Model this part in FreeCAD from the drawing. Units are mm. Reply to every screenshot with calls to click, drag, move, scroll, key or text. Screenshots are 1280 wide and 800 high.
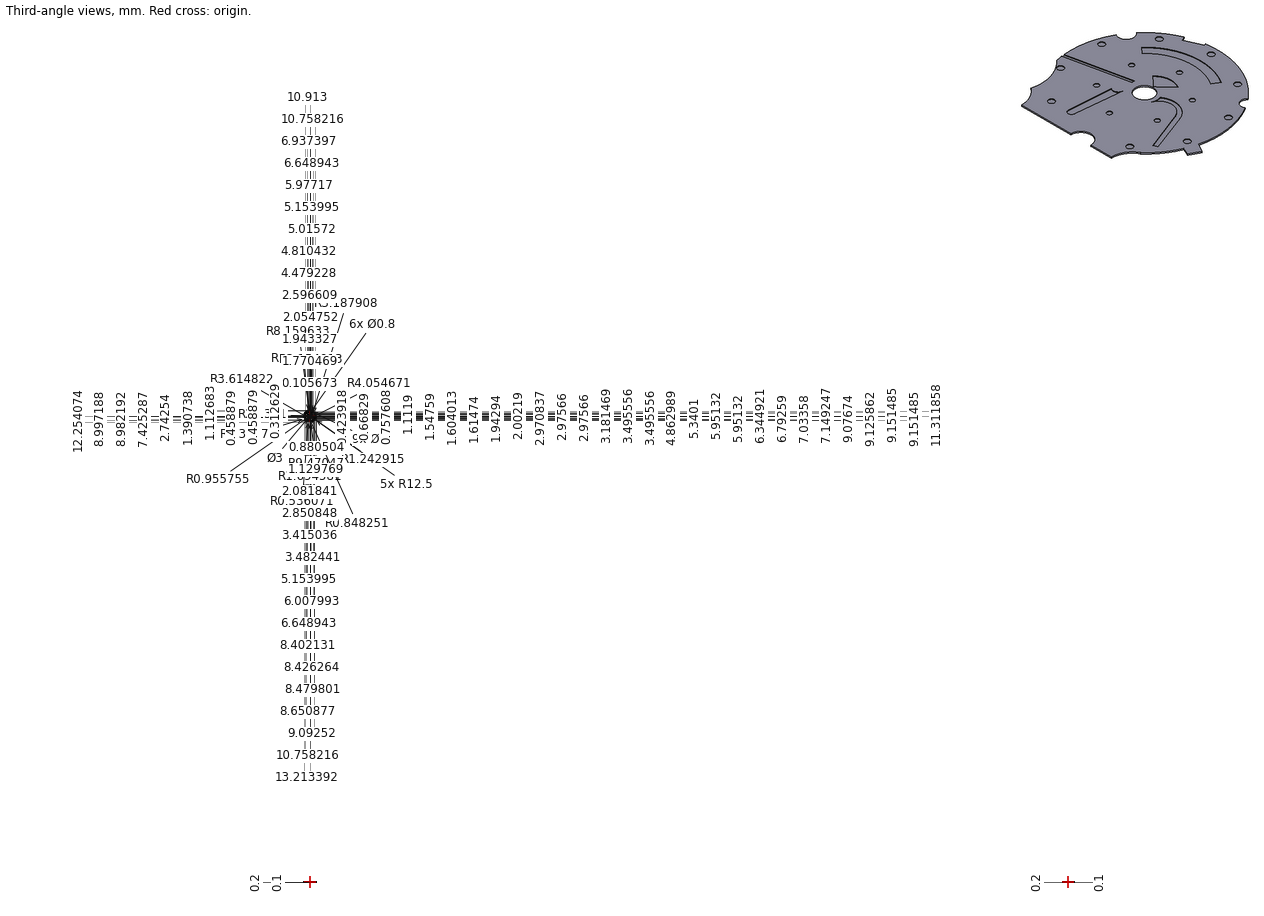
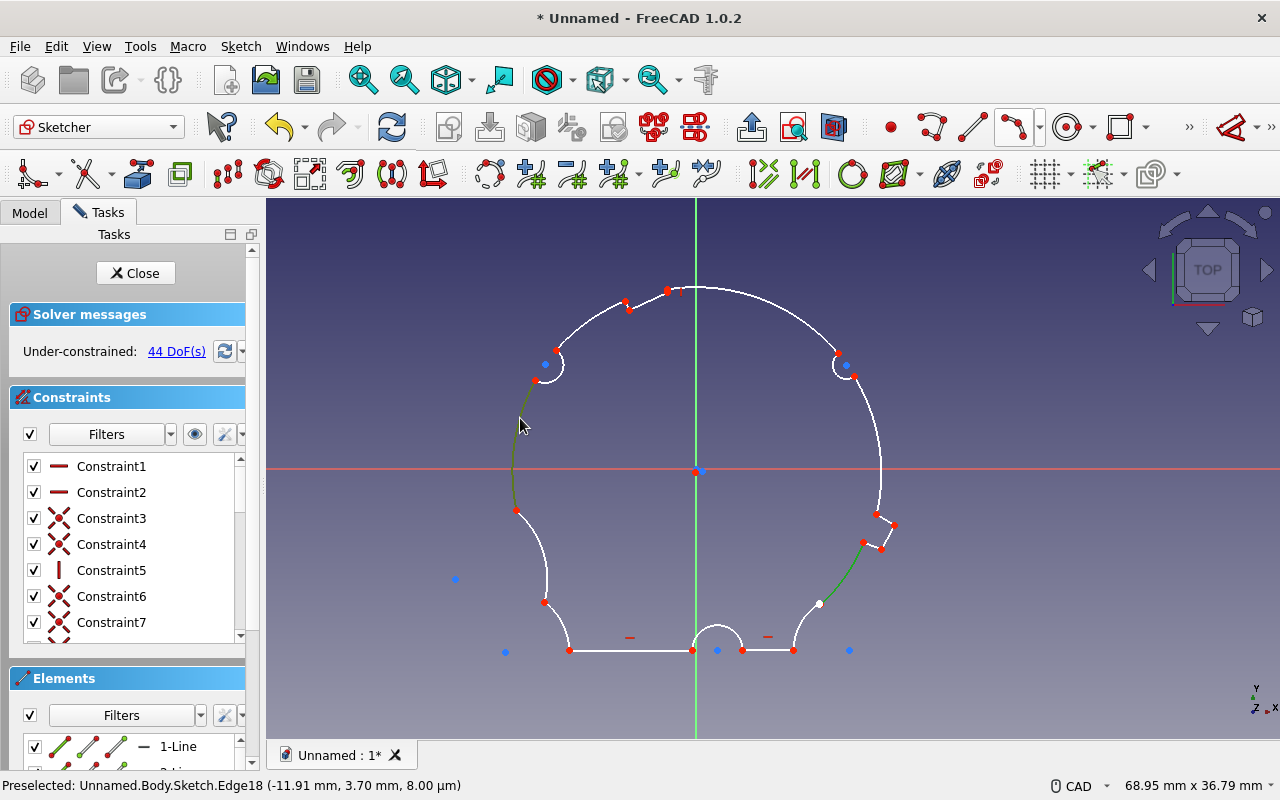
key(c)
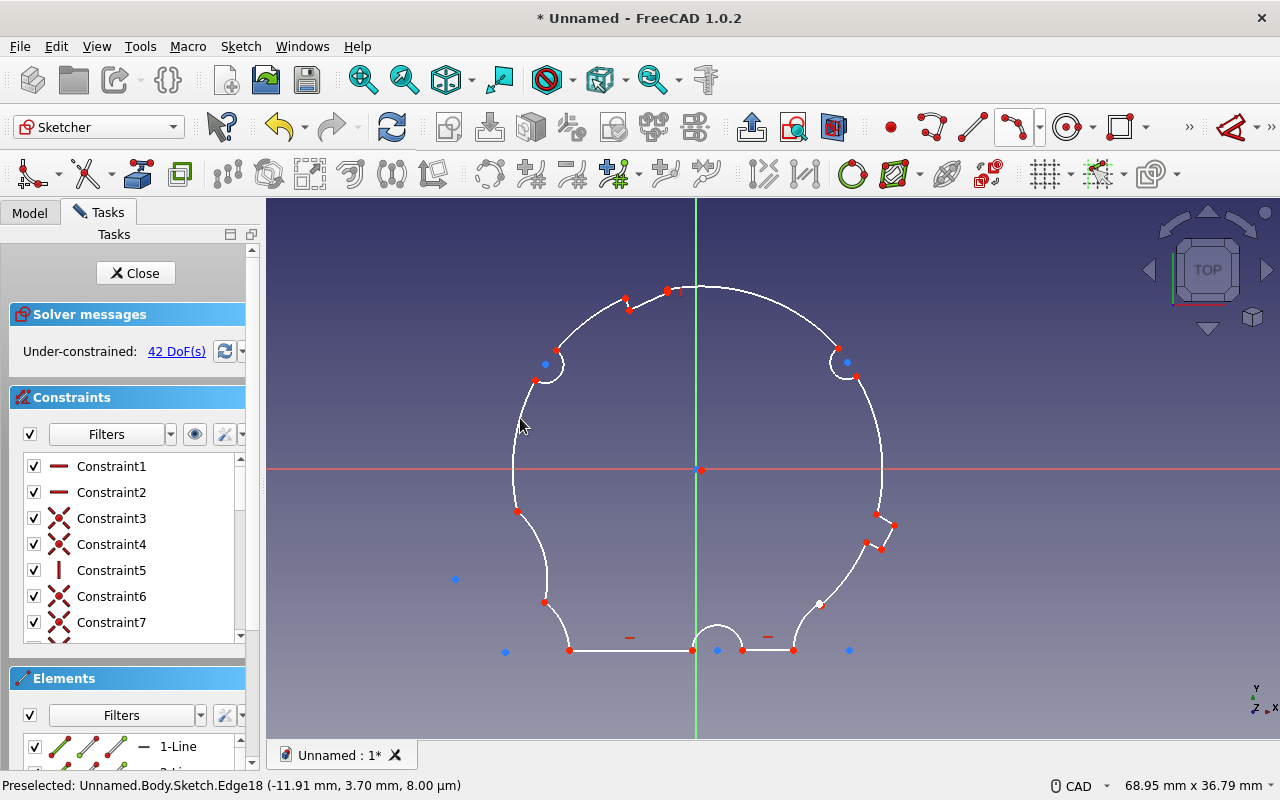
scroll(699, 470, up, 5)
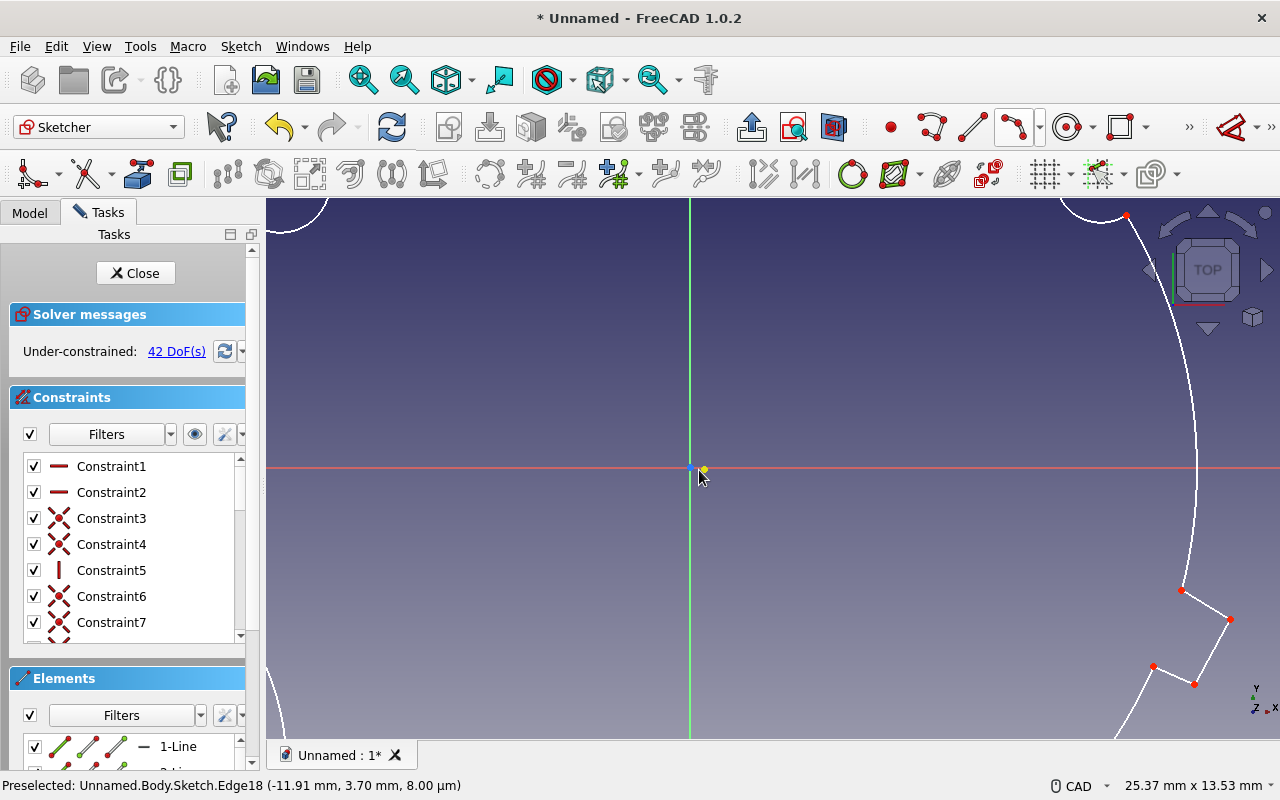
drag(680, 458, 715, 479)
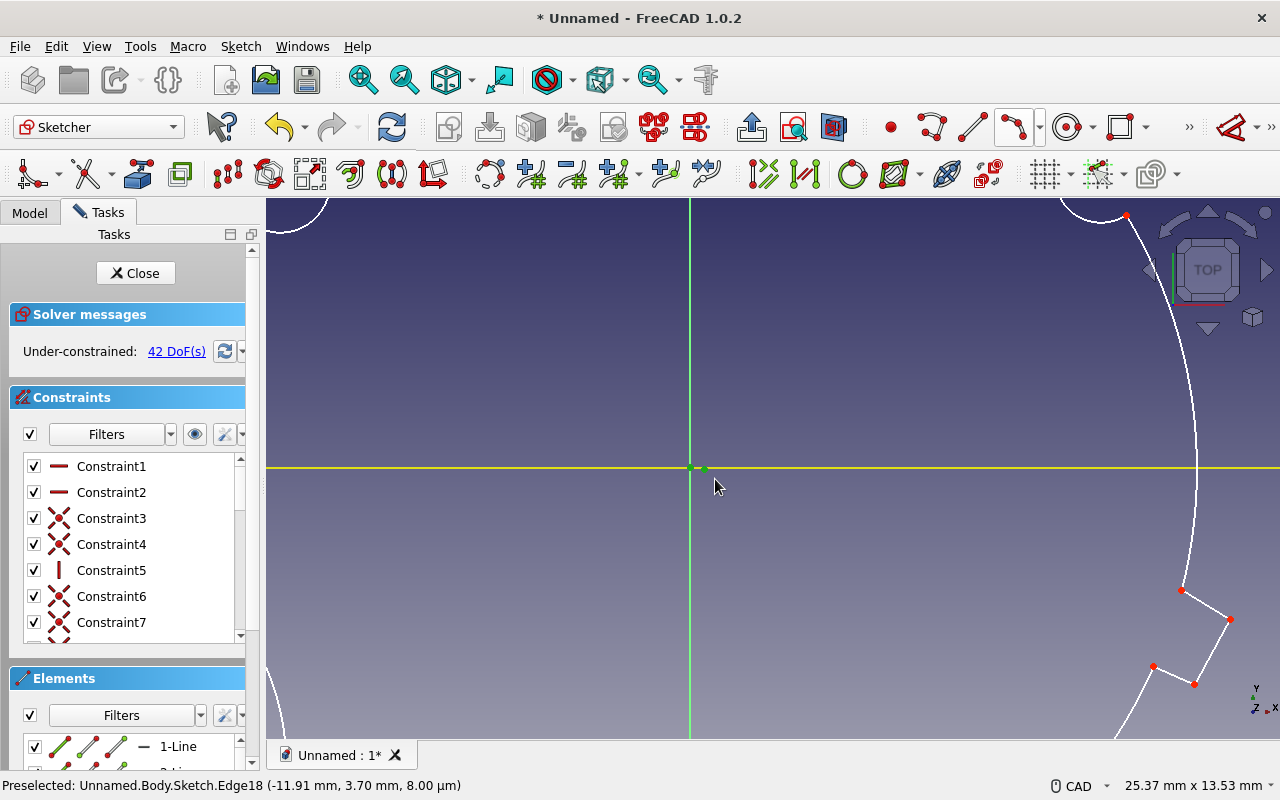
key(c)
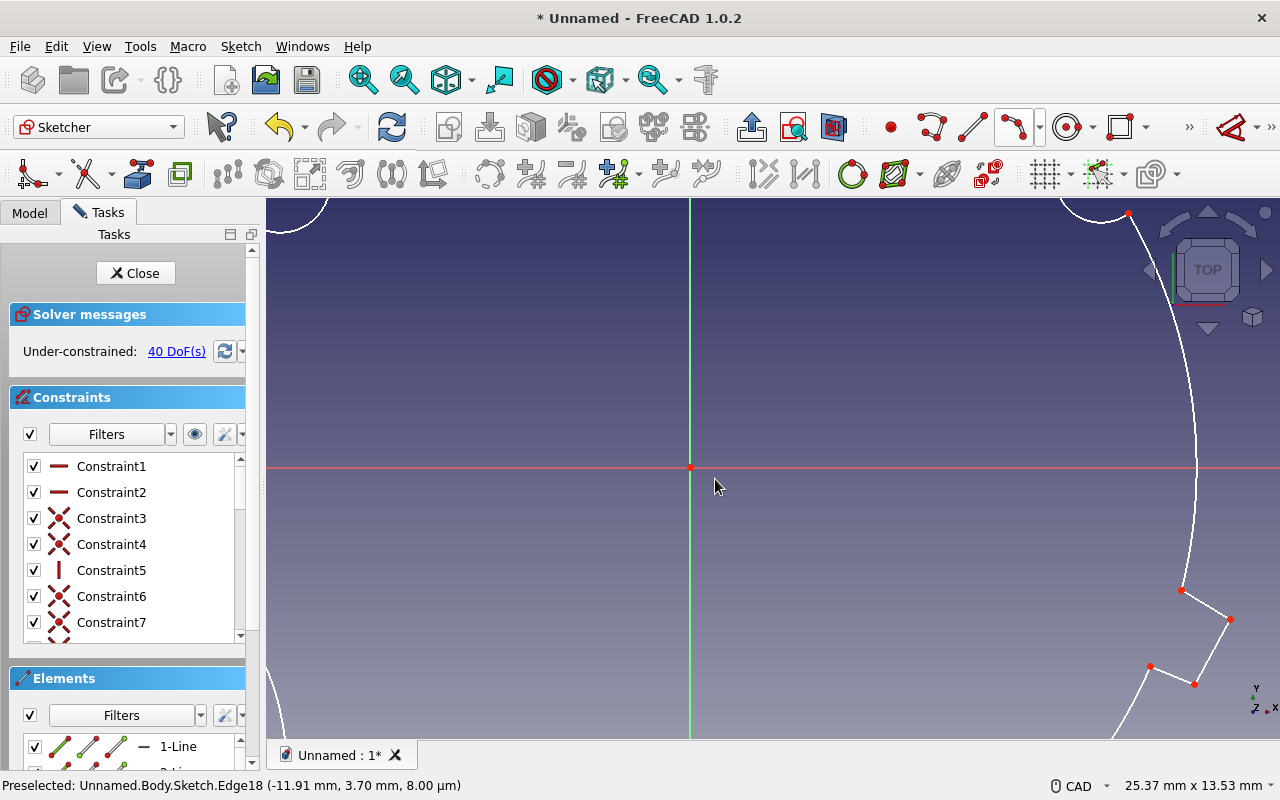
scroll(699, 470, down, 5)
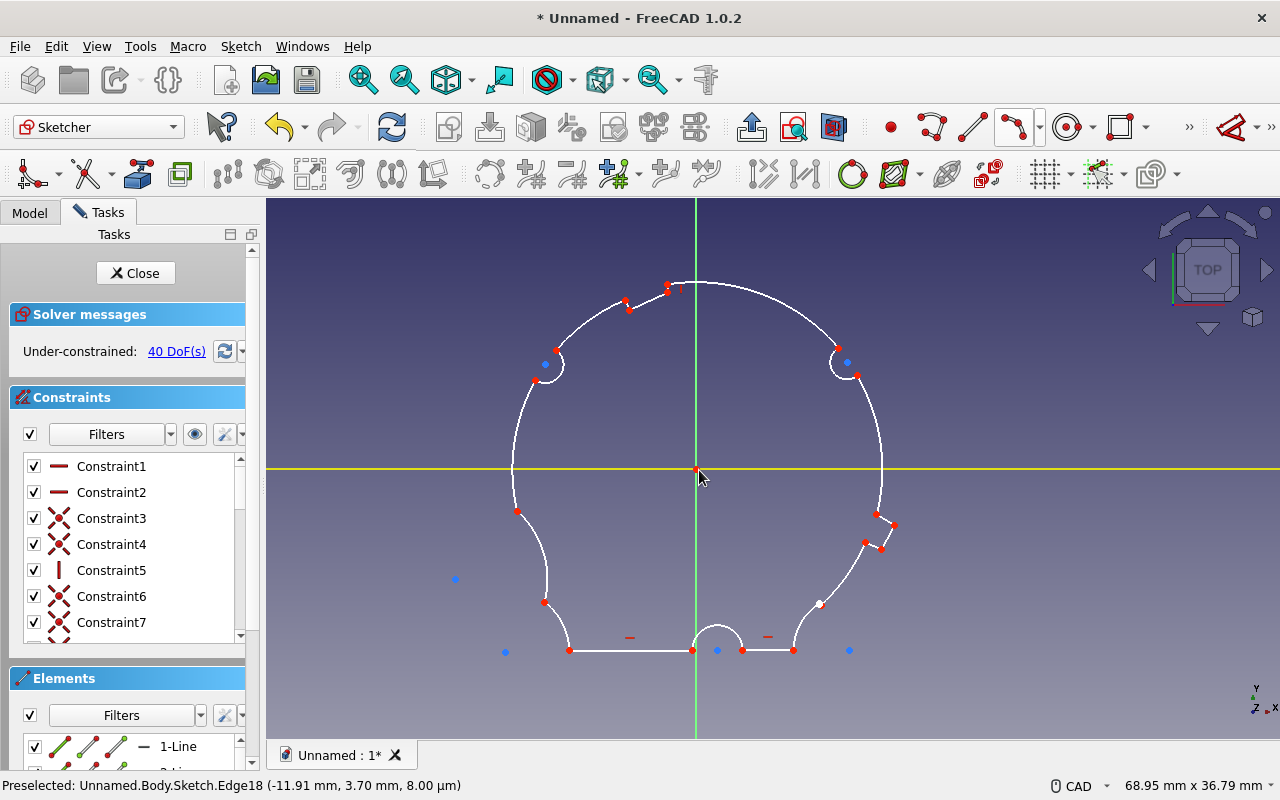
click(837, 588)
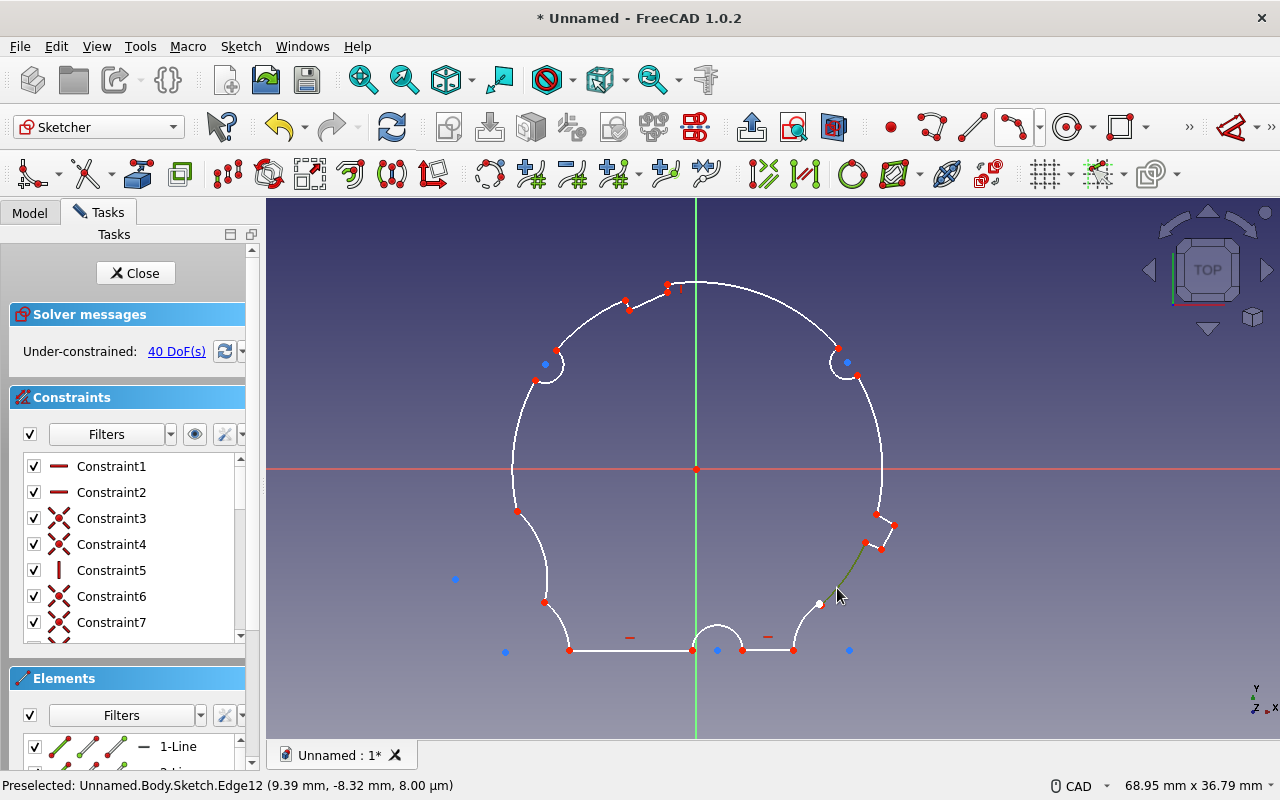
click(882, 472)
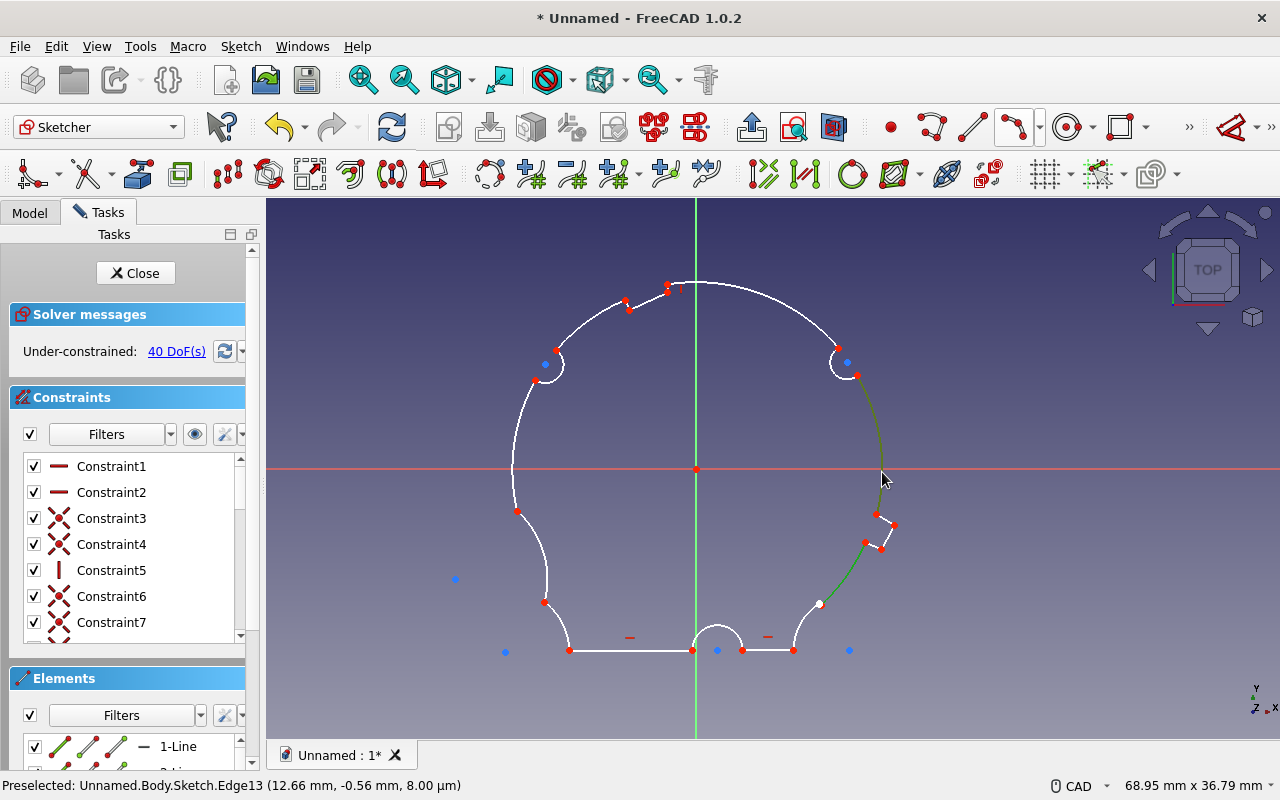
click(795, 311)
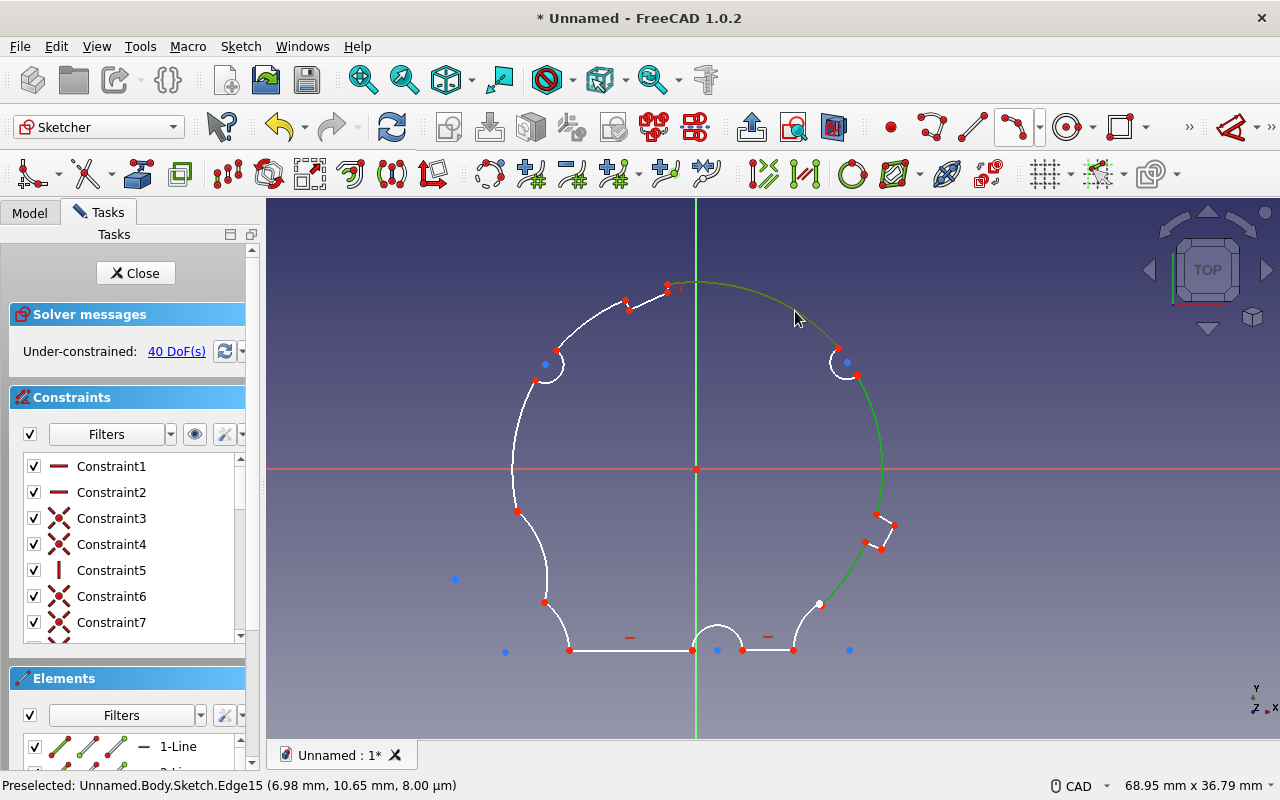
click(602, 312)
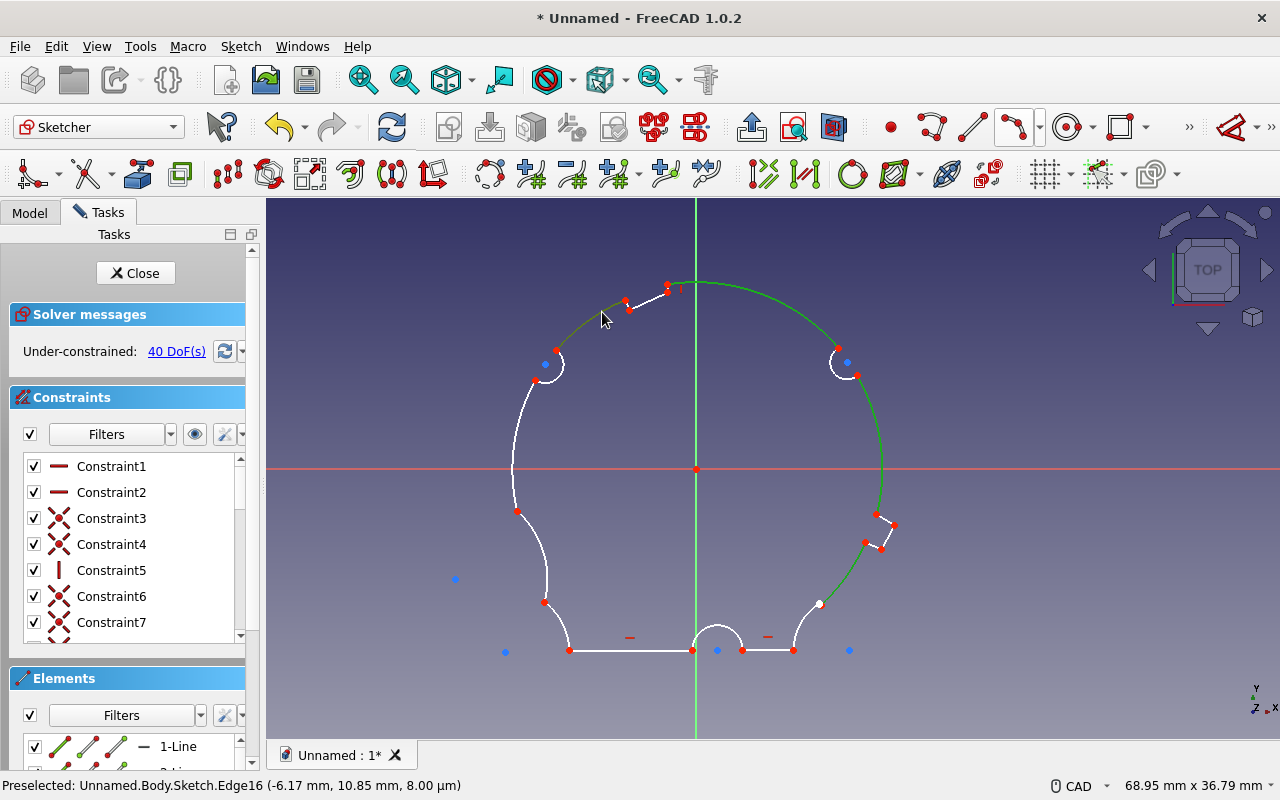
click(520, 418)